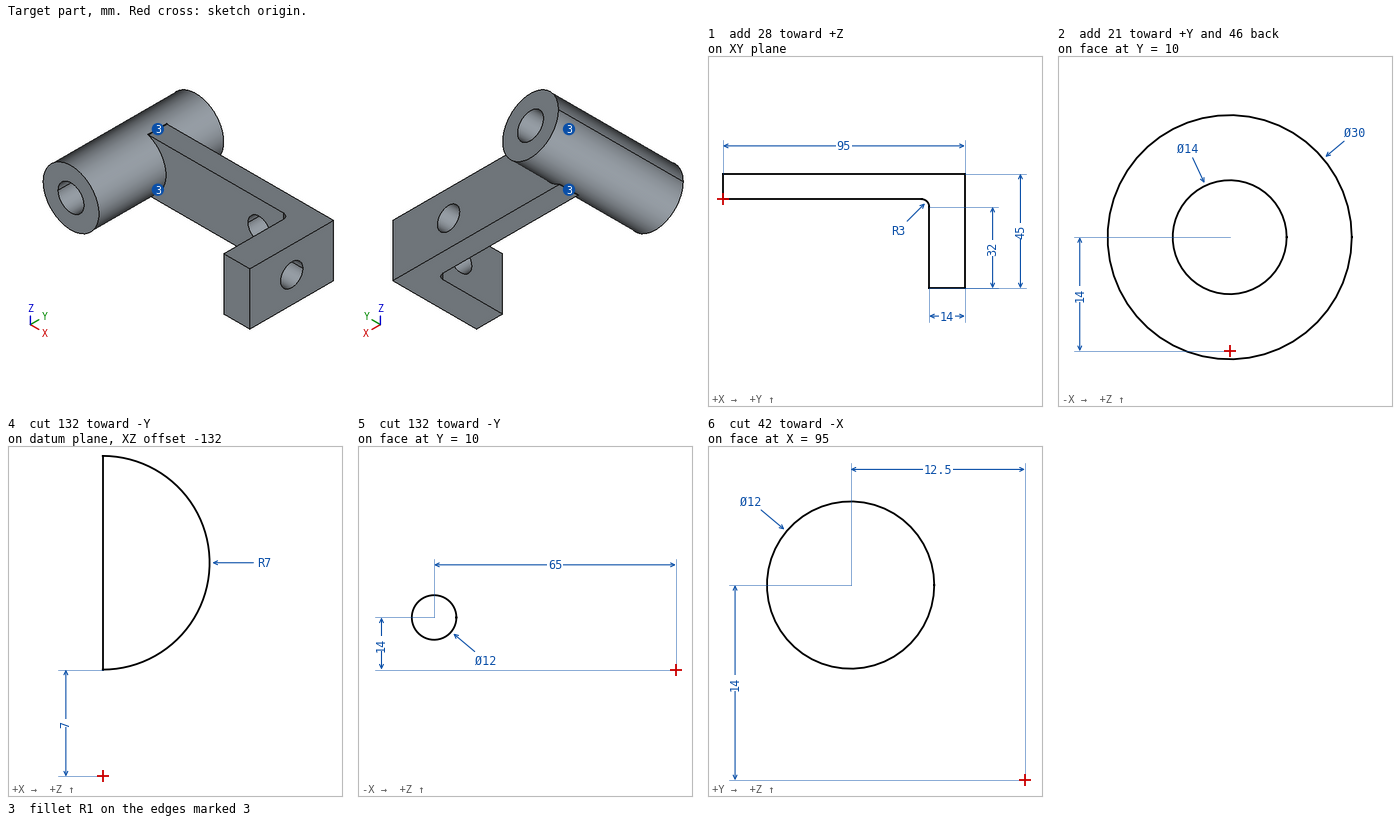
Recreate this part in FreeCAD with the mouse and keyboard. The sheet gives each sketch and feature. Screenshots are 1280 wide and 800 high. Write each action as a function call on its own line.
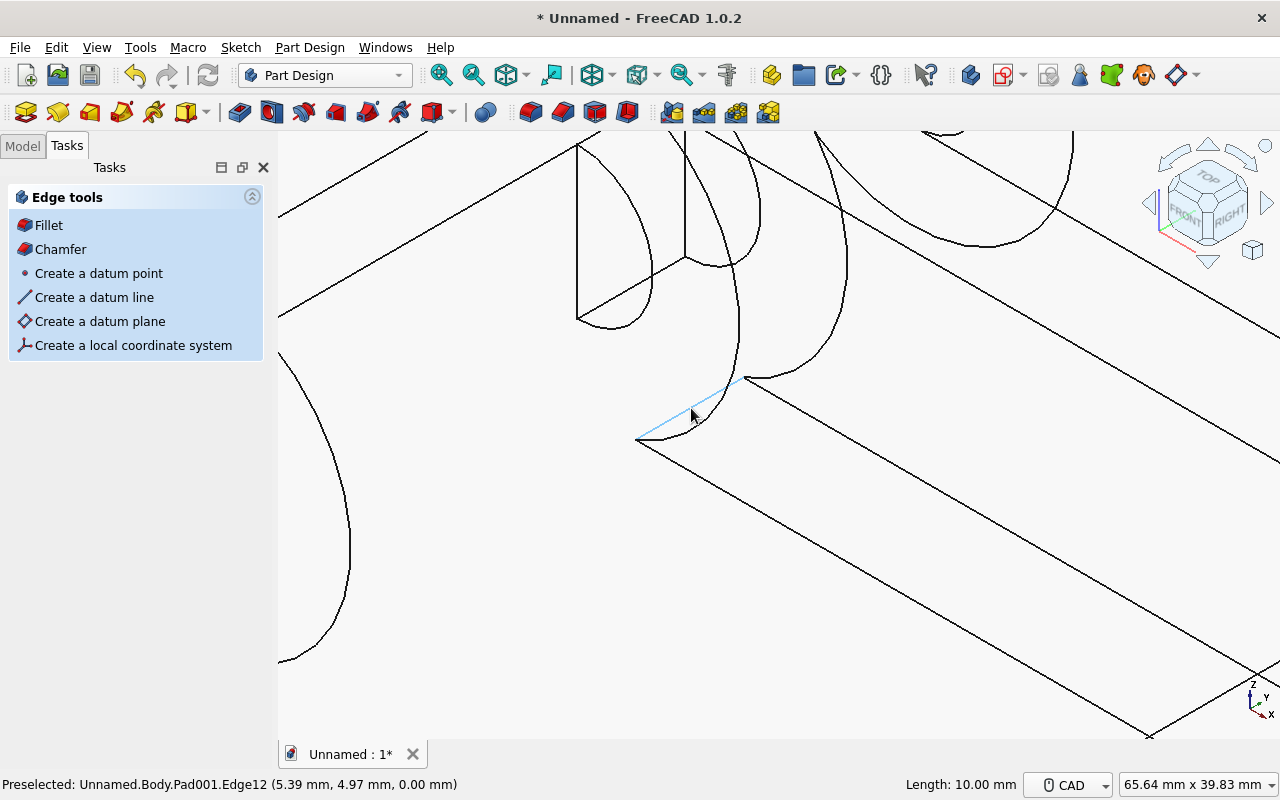
click(690, 408, ctrl)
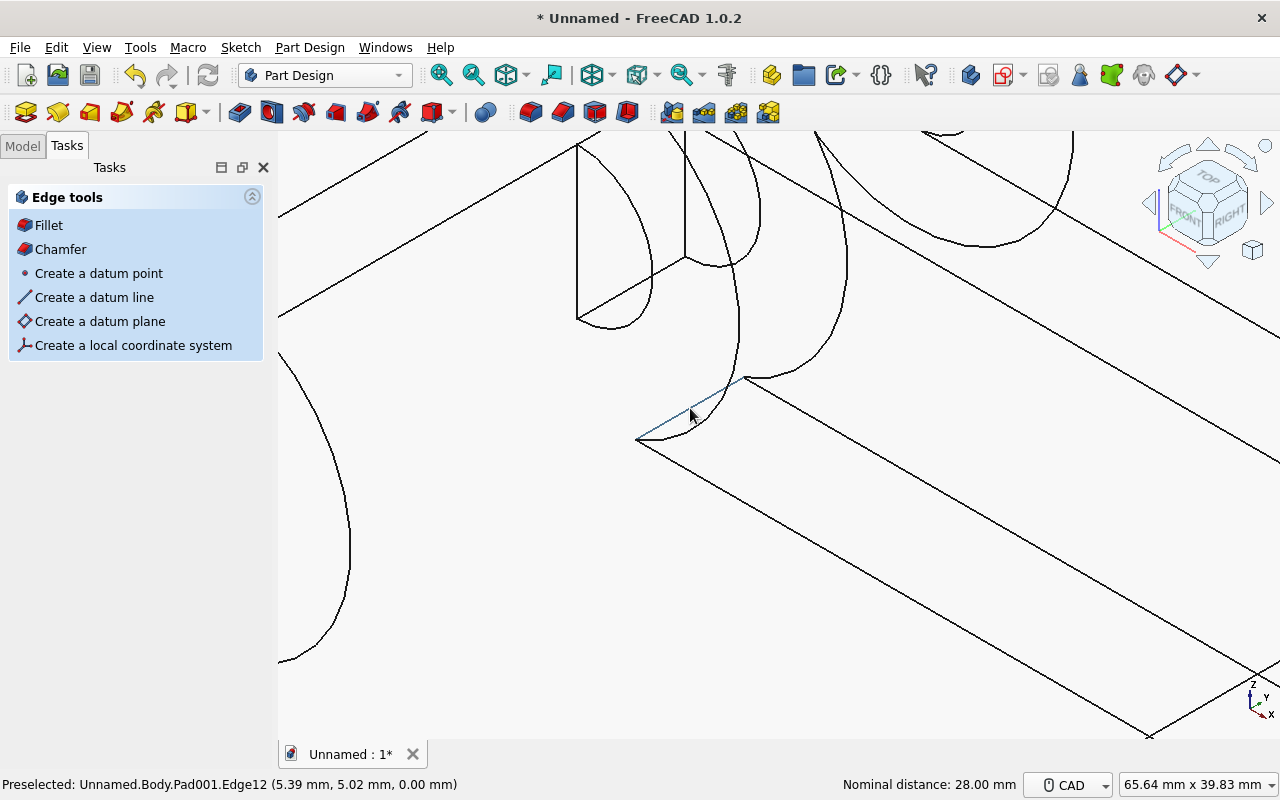
key(v)
key(1)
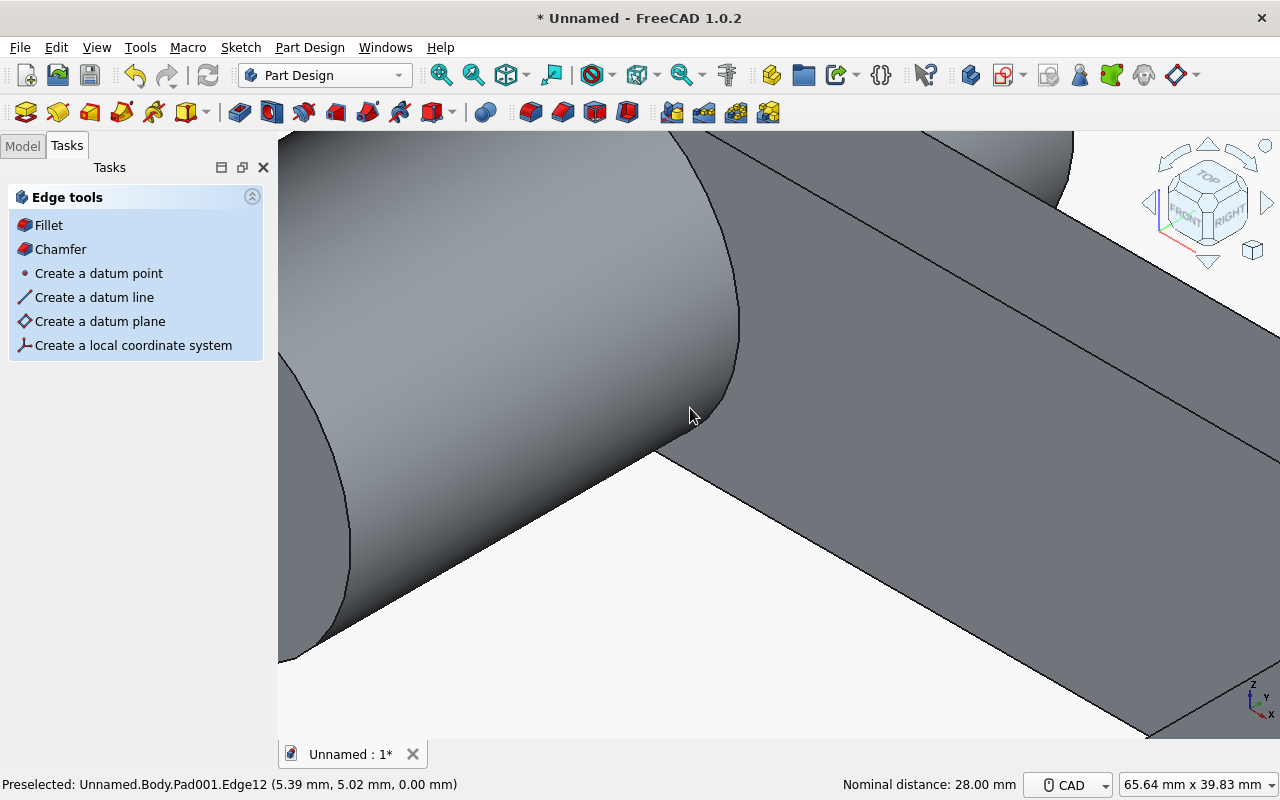
click(532, 112)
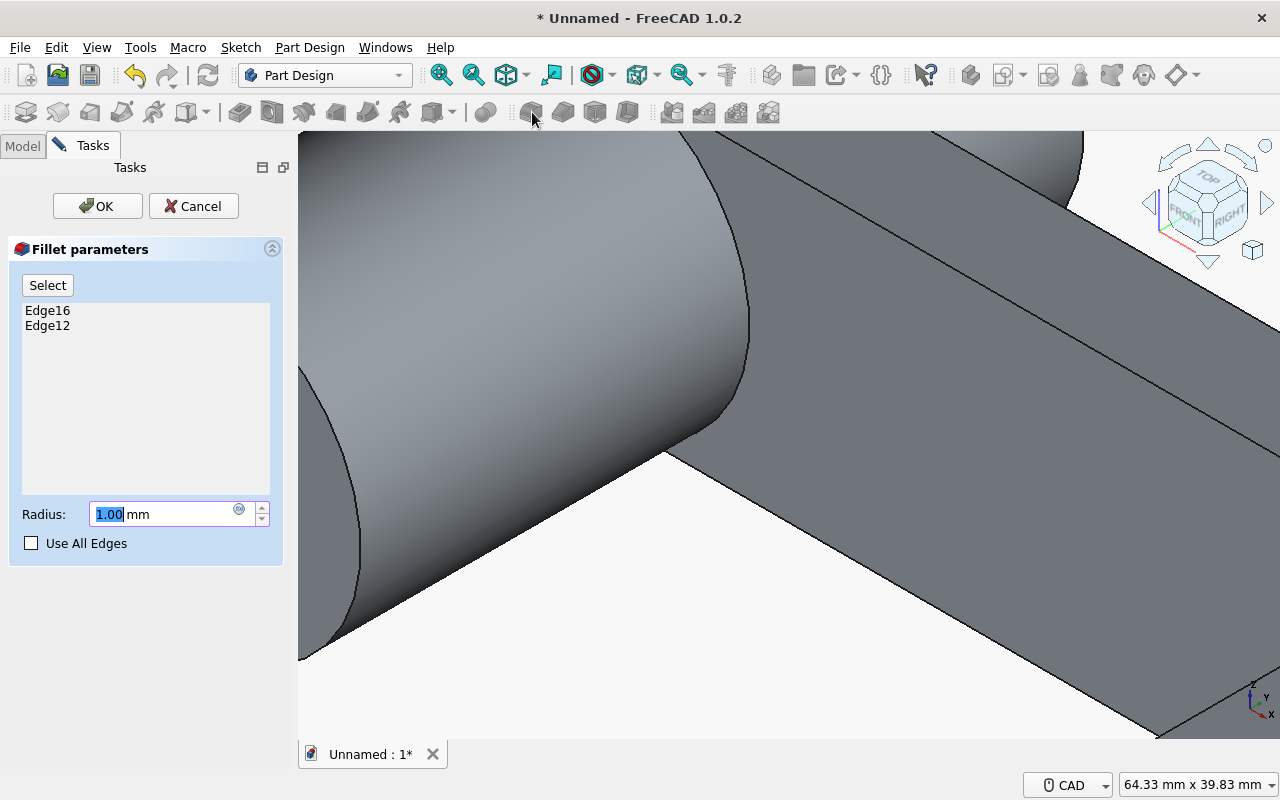
text(1)
key(Tab)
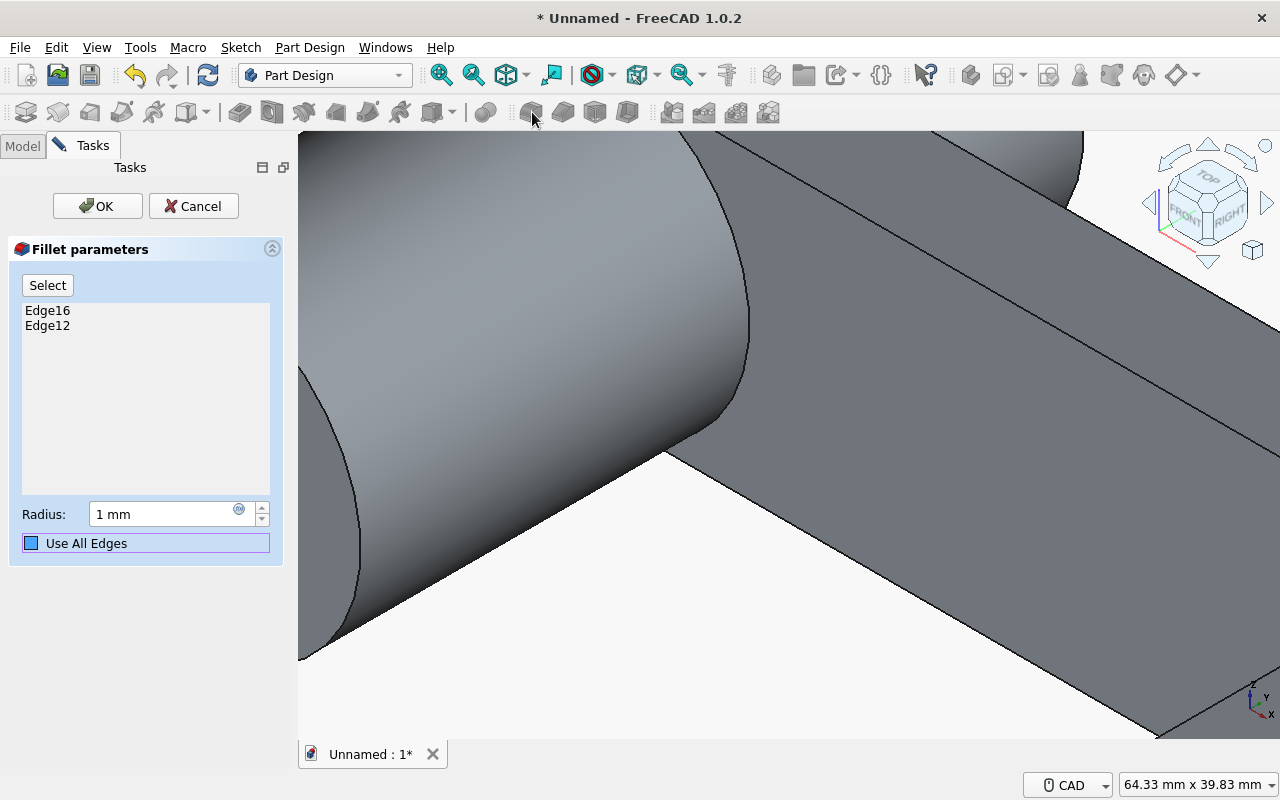
click(98, 206)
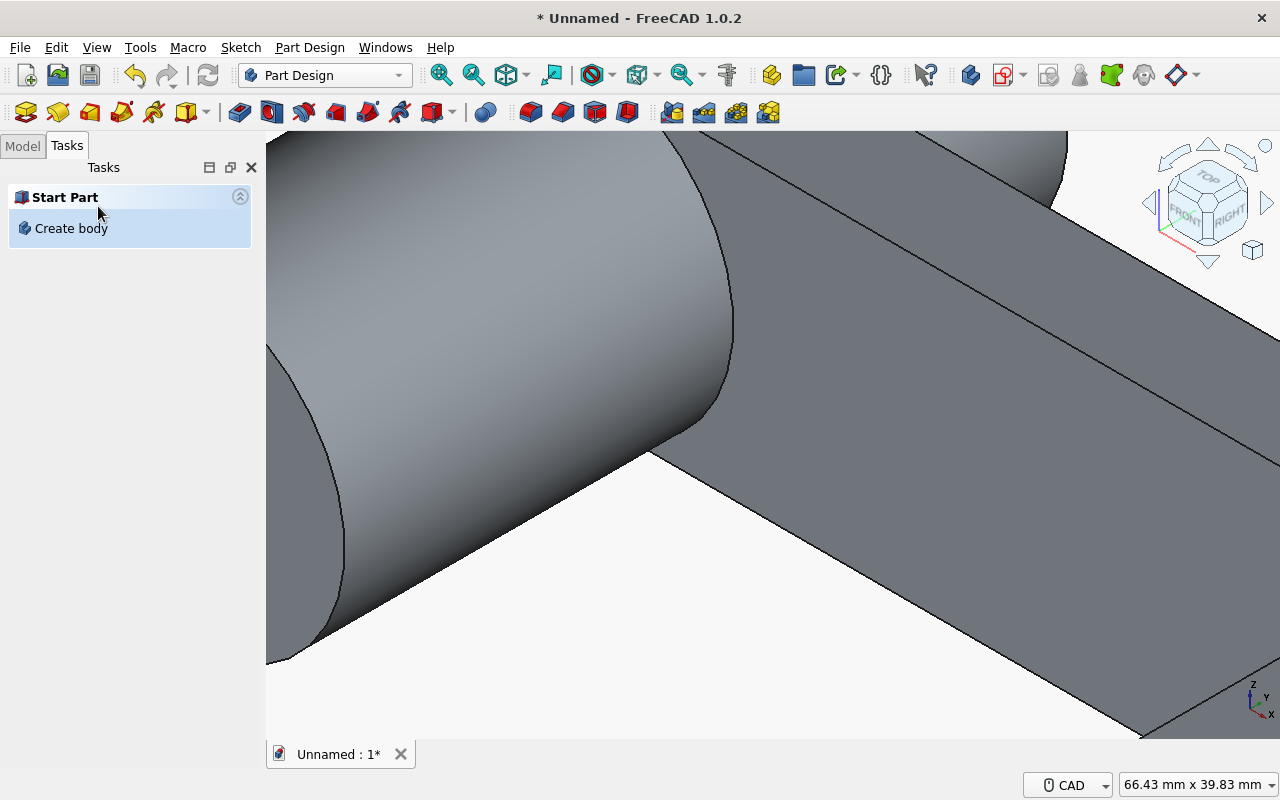
click(442, 76)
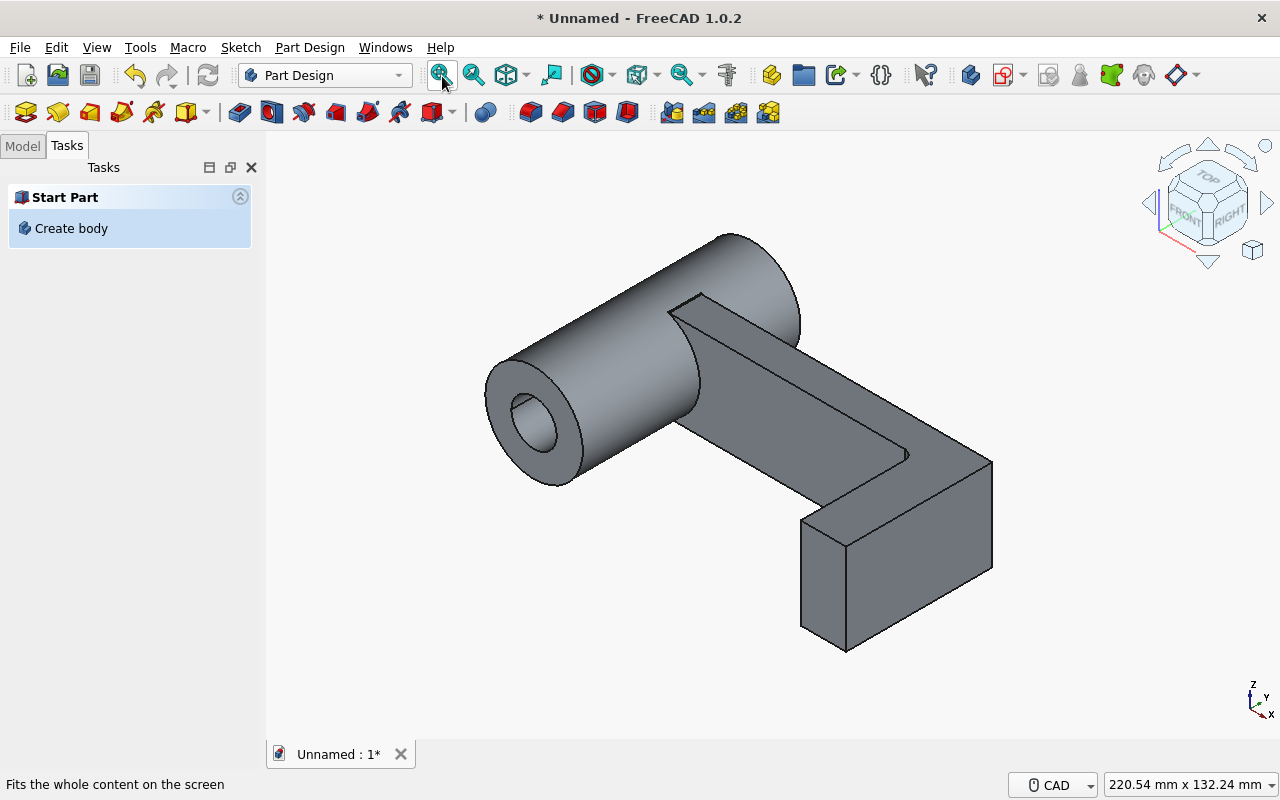
click(23, 145)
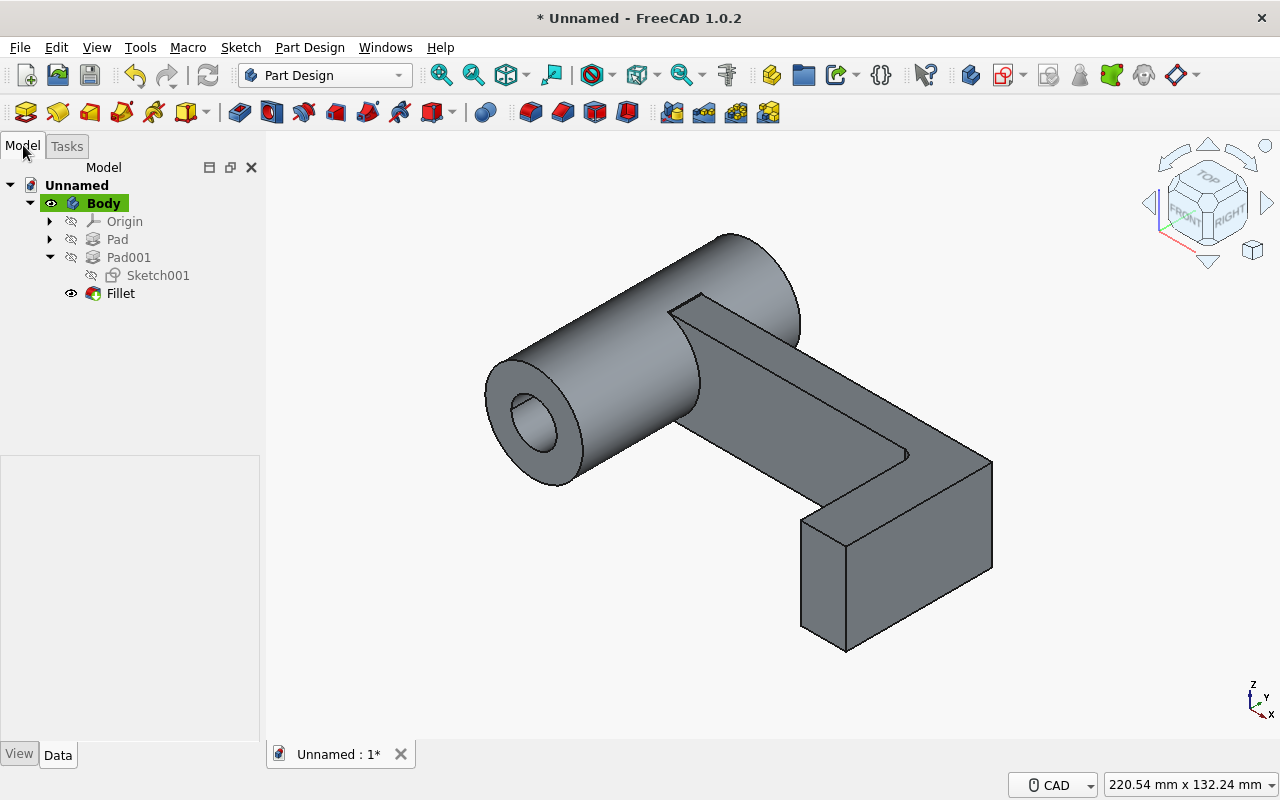
click(50, 221)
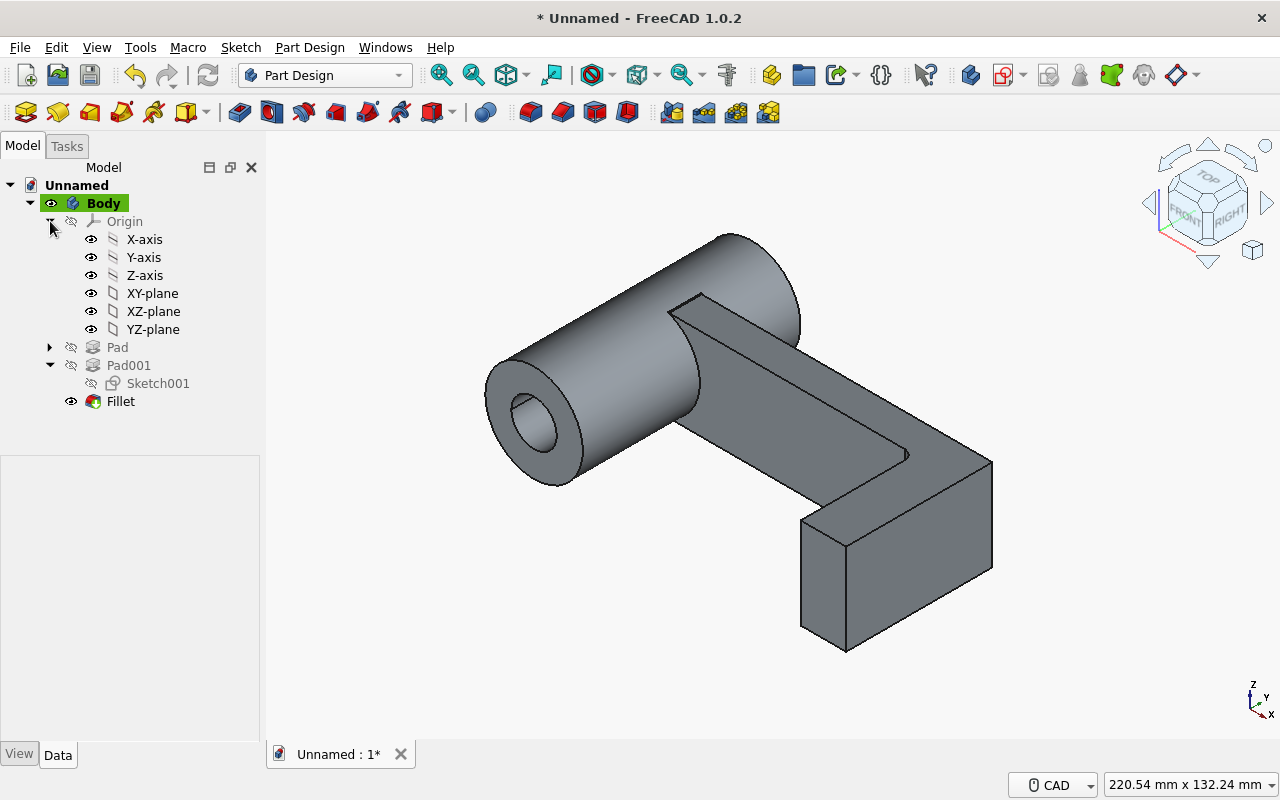
click(136, 311)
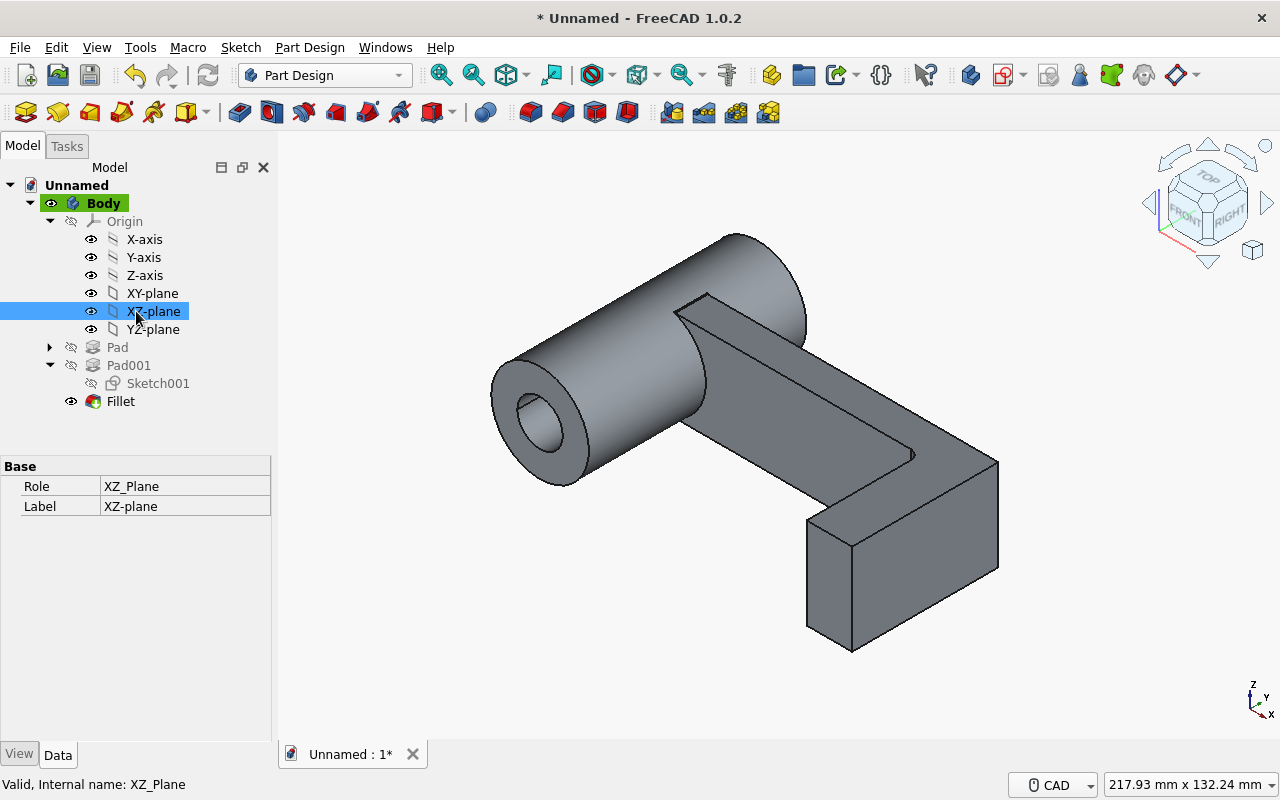
click(1176, 76)